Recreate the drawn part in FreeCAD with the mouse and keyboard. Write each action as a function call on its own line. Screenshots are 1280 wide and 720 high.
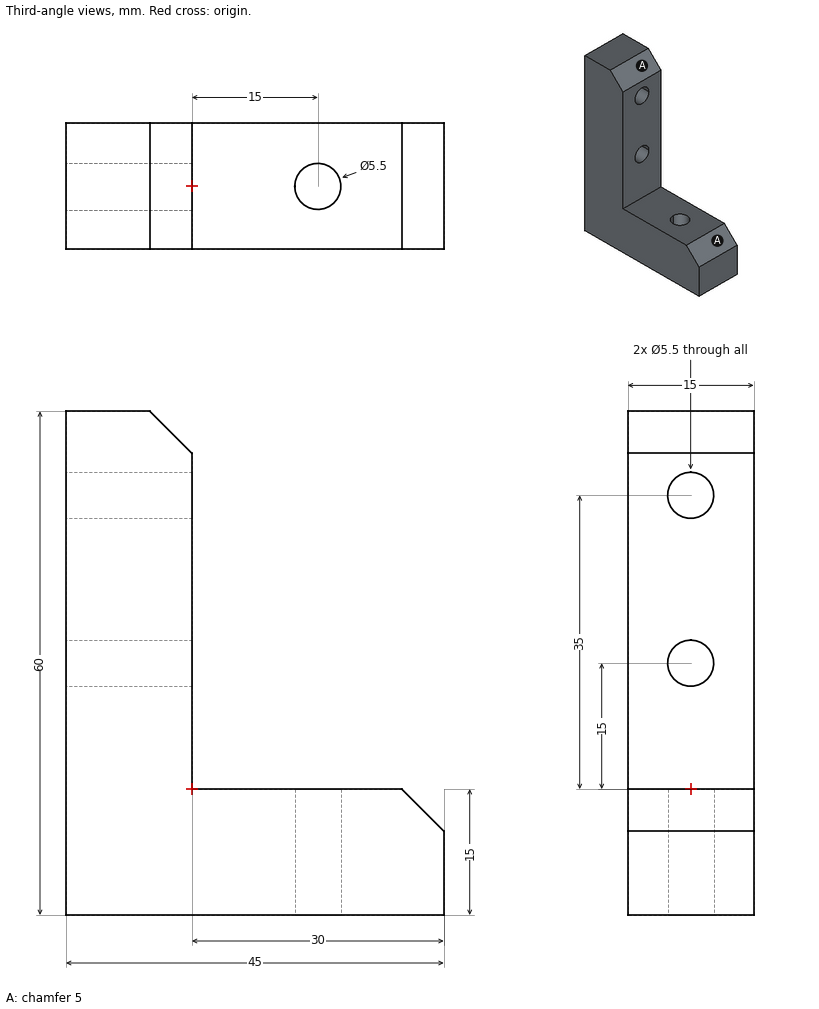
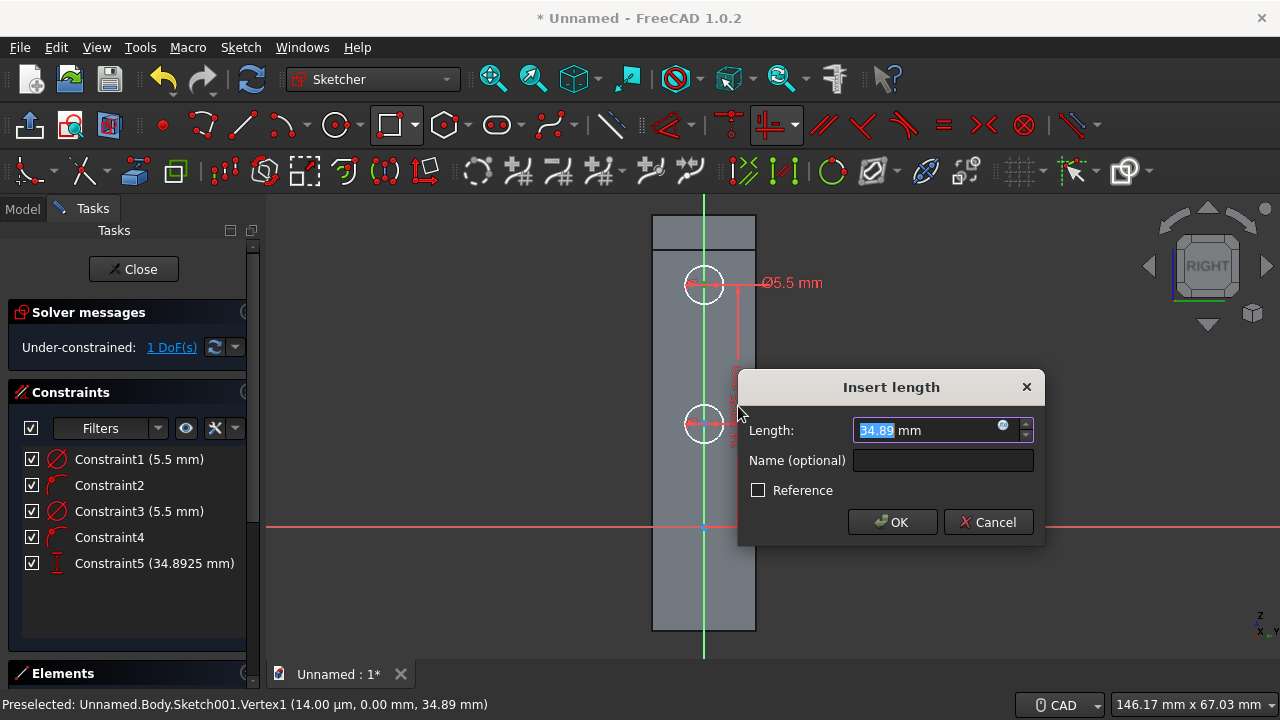
text(35)
key(Return)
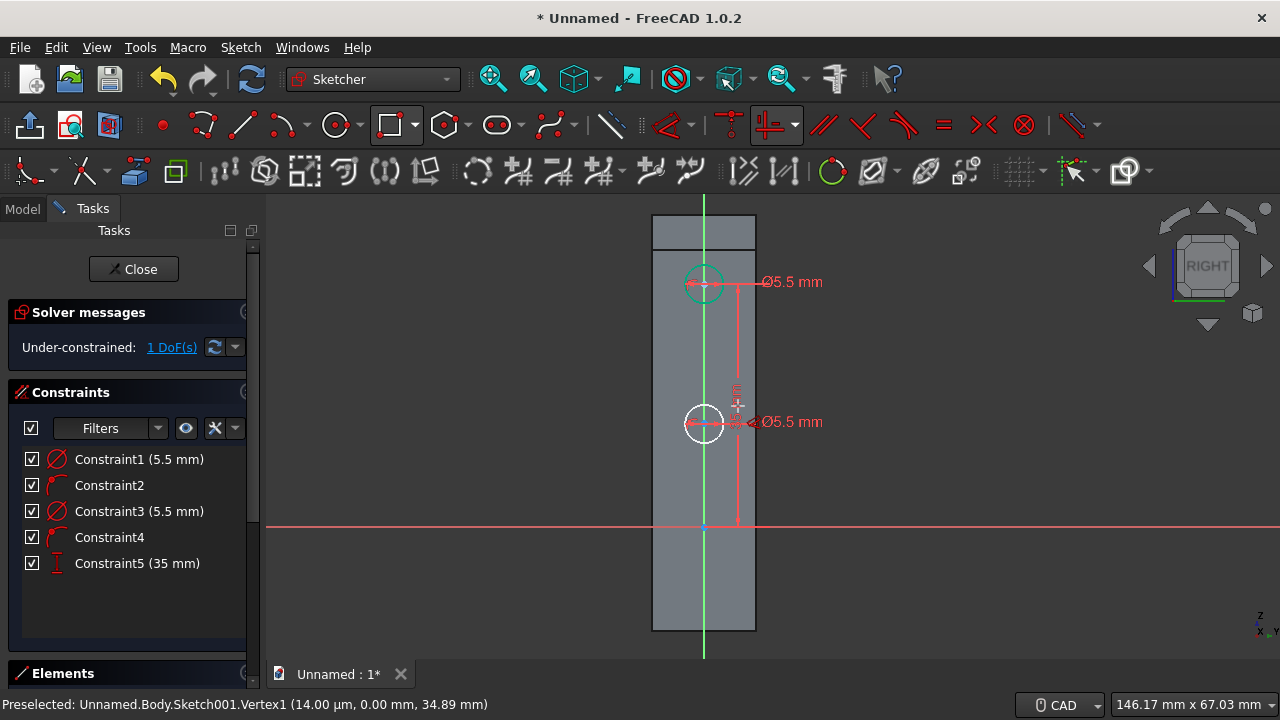
click(704, 424)
click(738, 476)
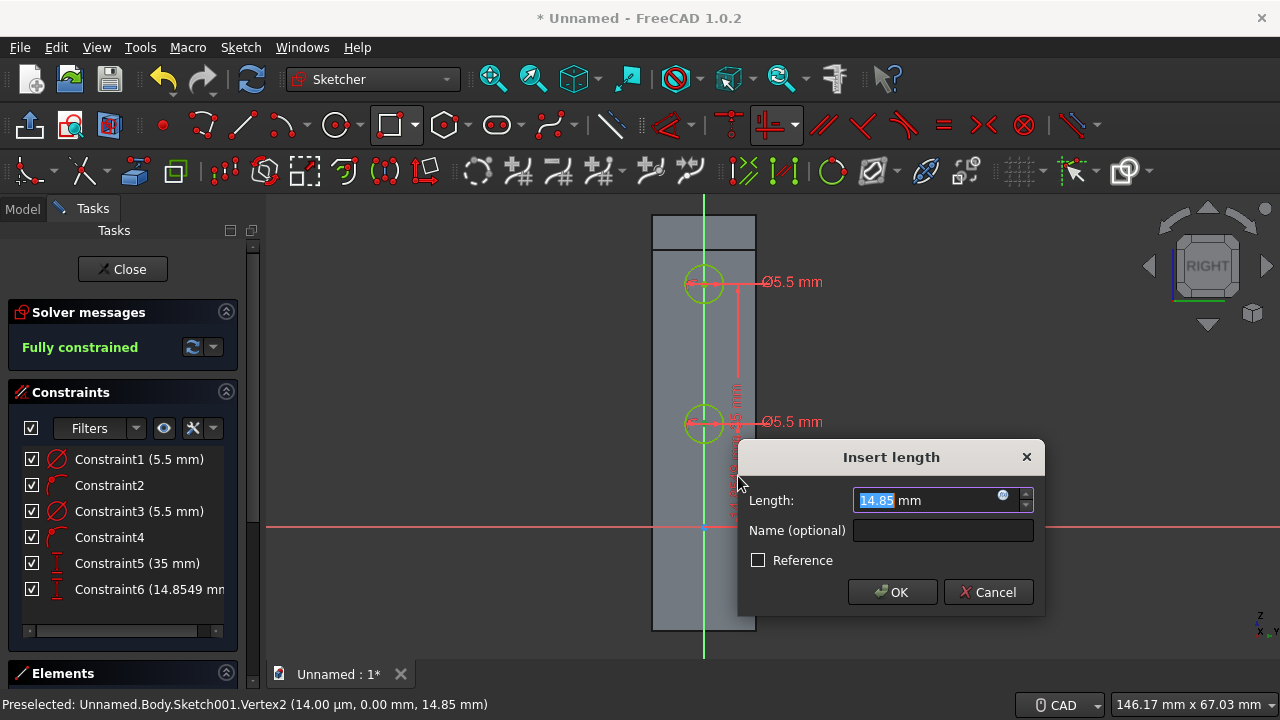
text(15)
key(Return)
key(Escape)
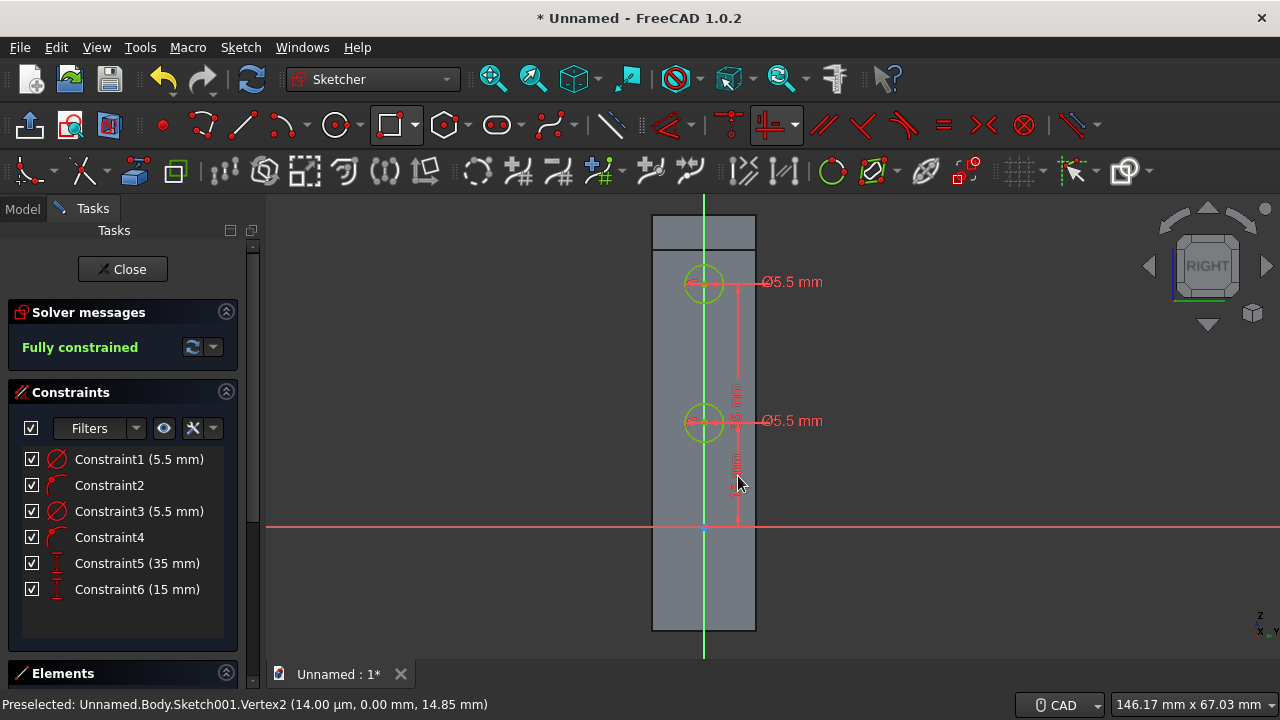
click(123, 269)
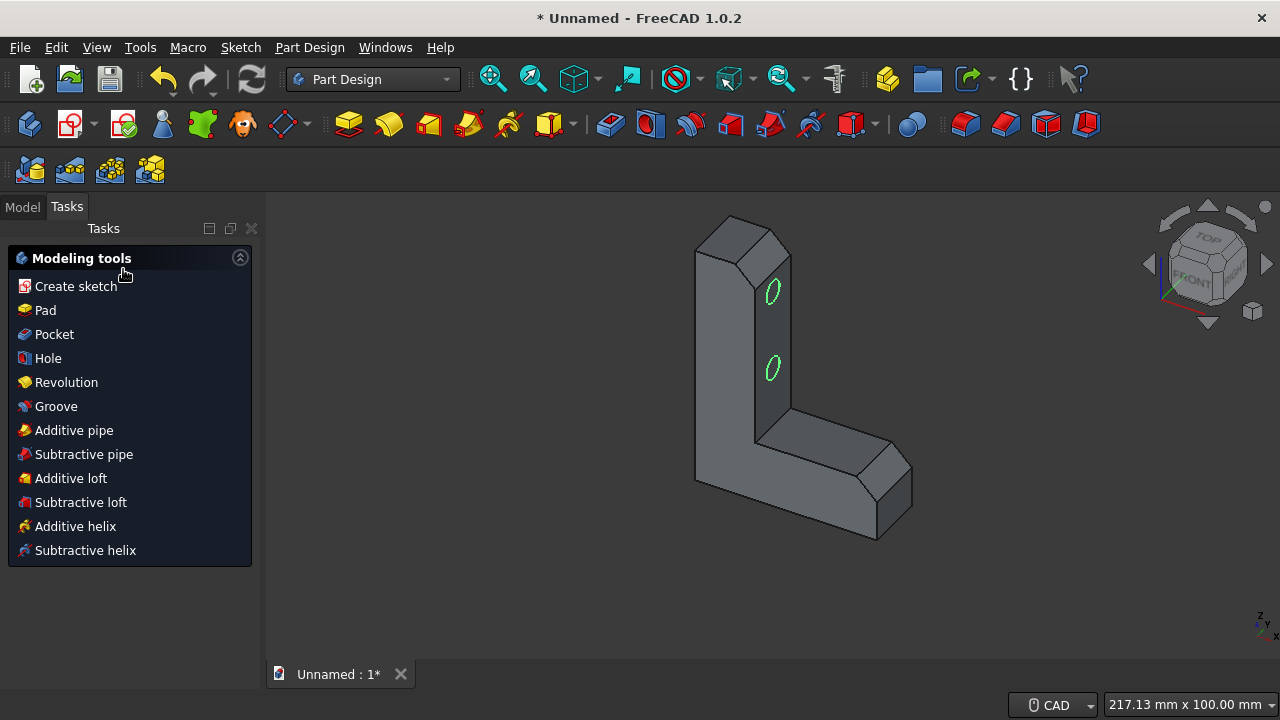
click(652, 124)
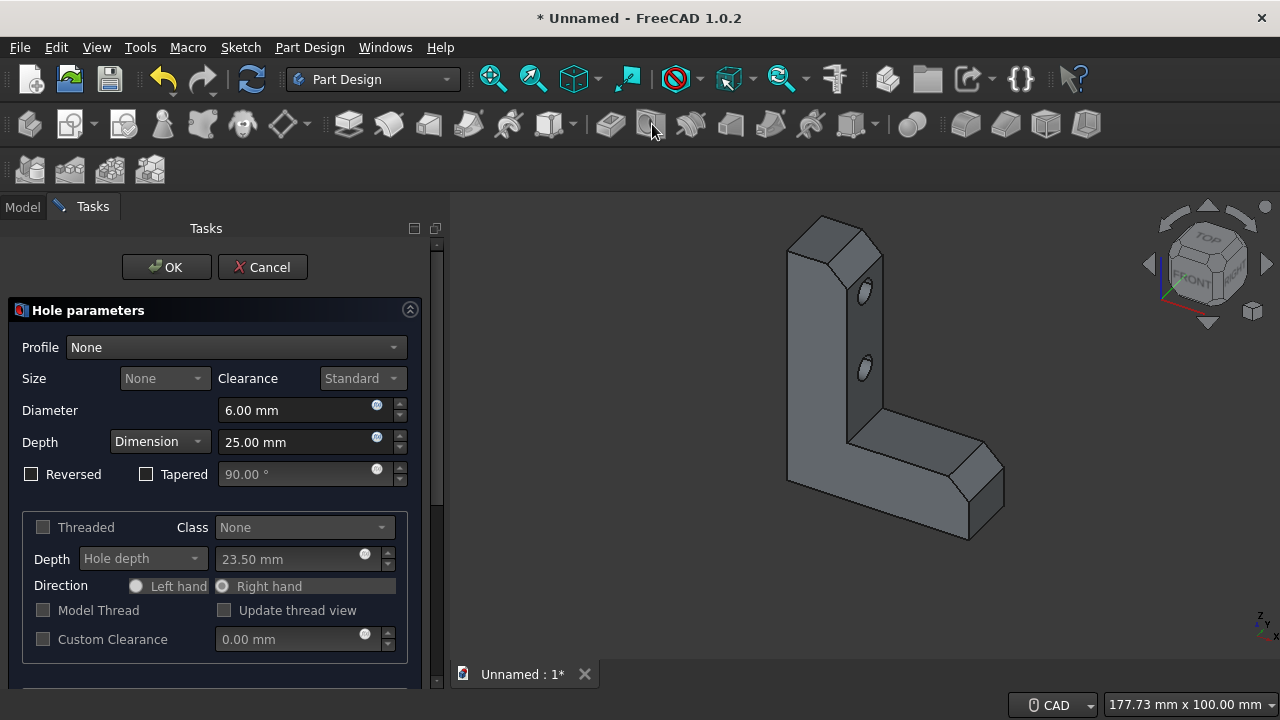
triple_click(305, 410)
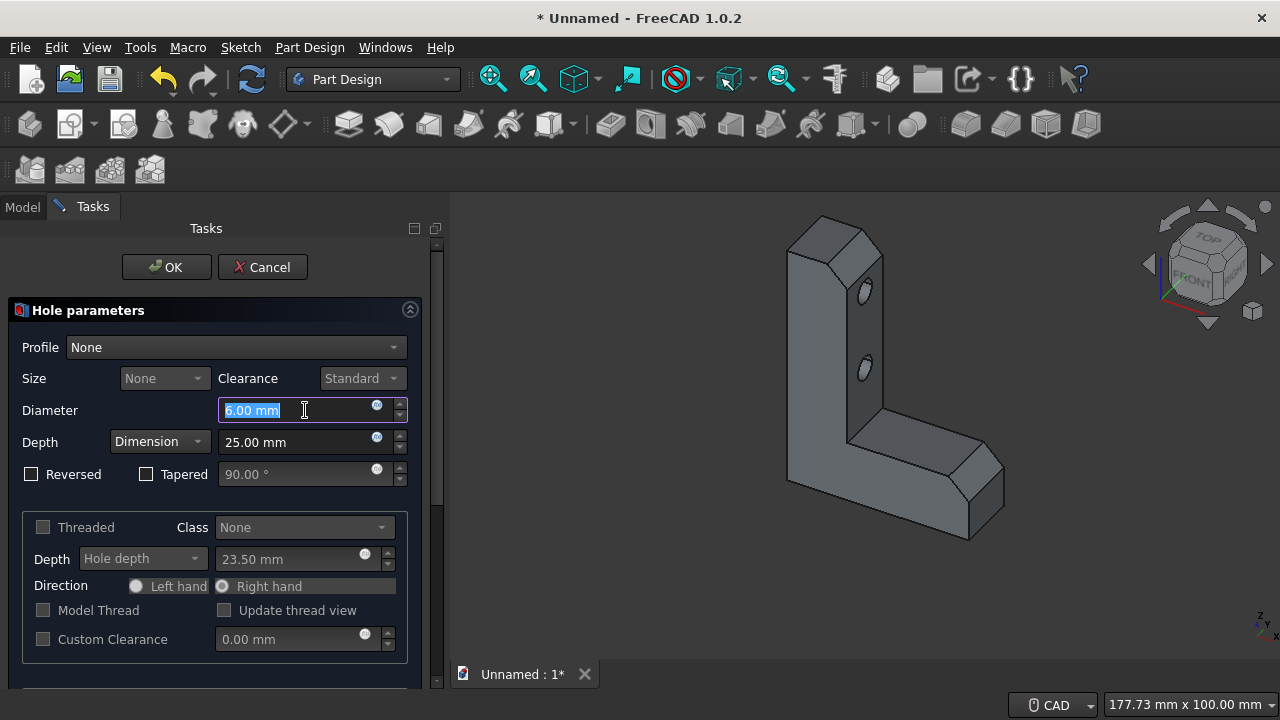
text(5.5)
key(Tab)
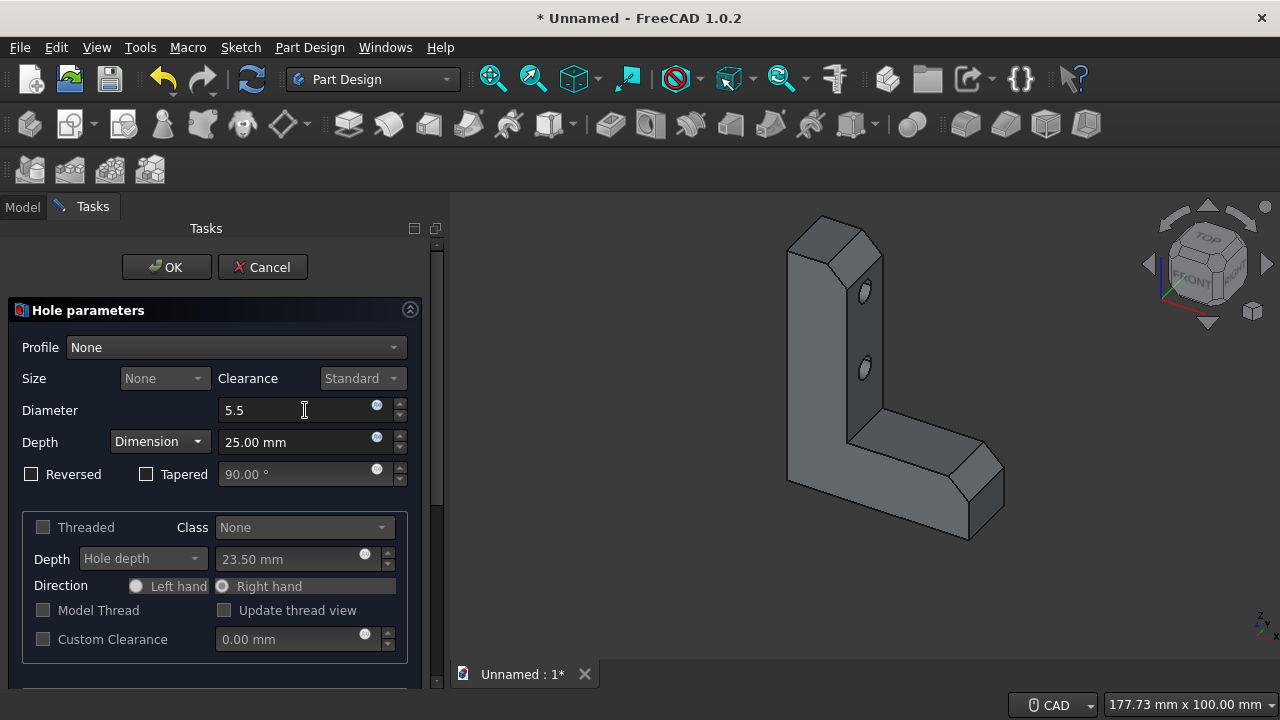
click(161, 442)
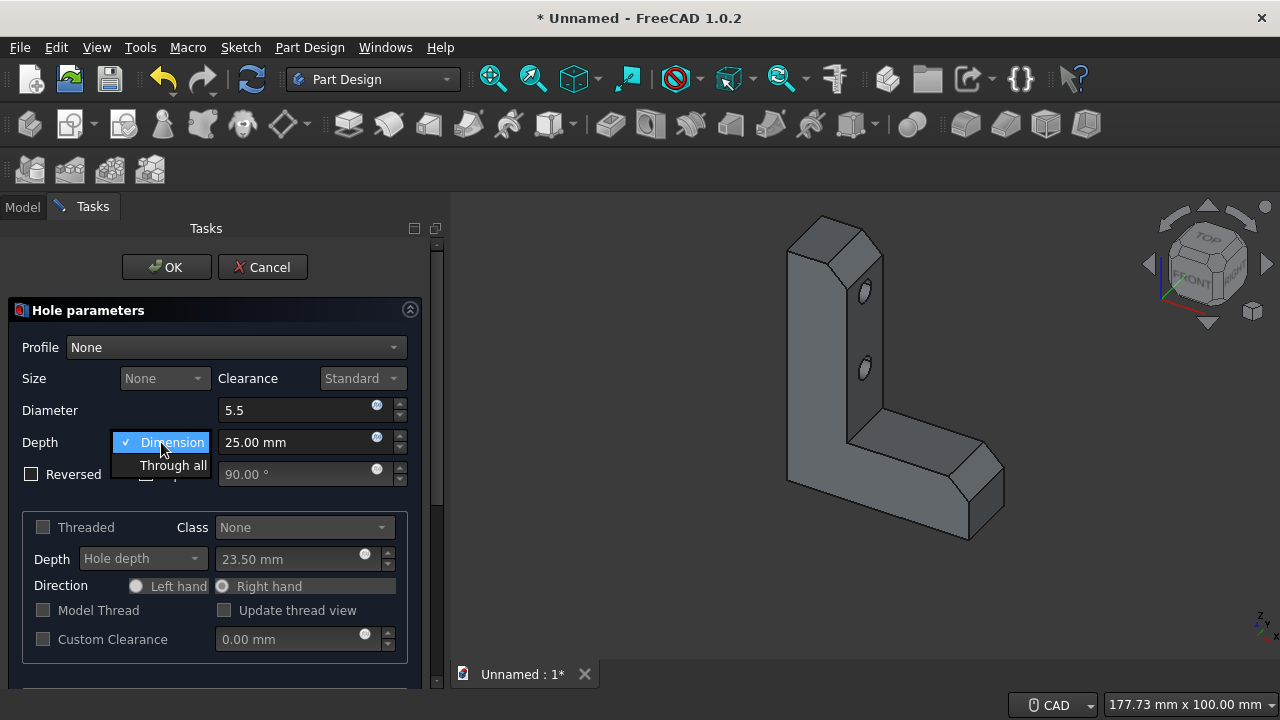
click(160, 466)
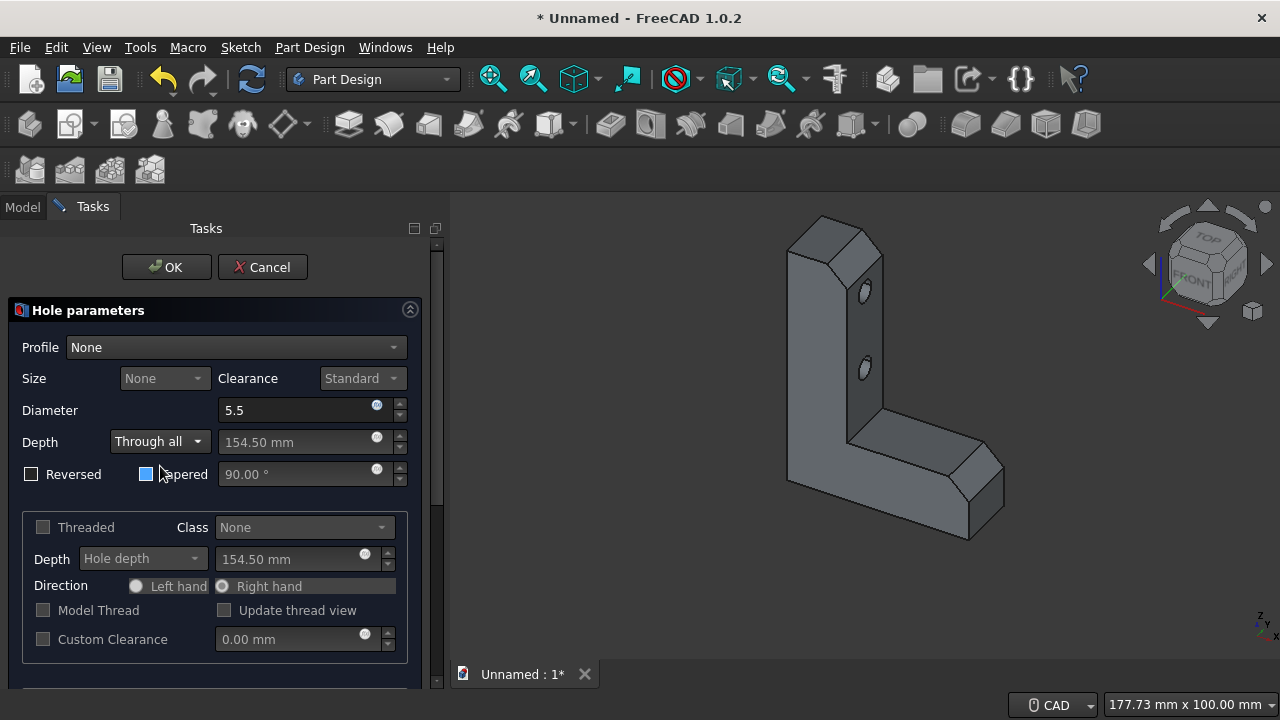
click(167, 267)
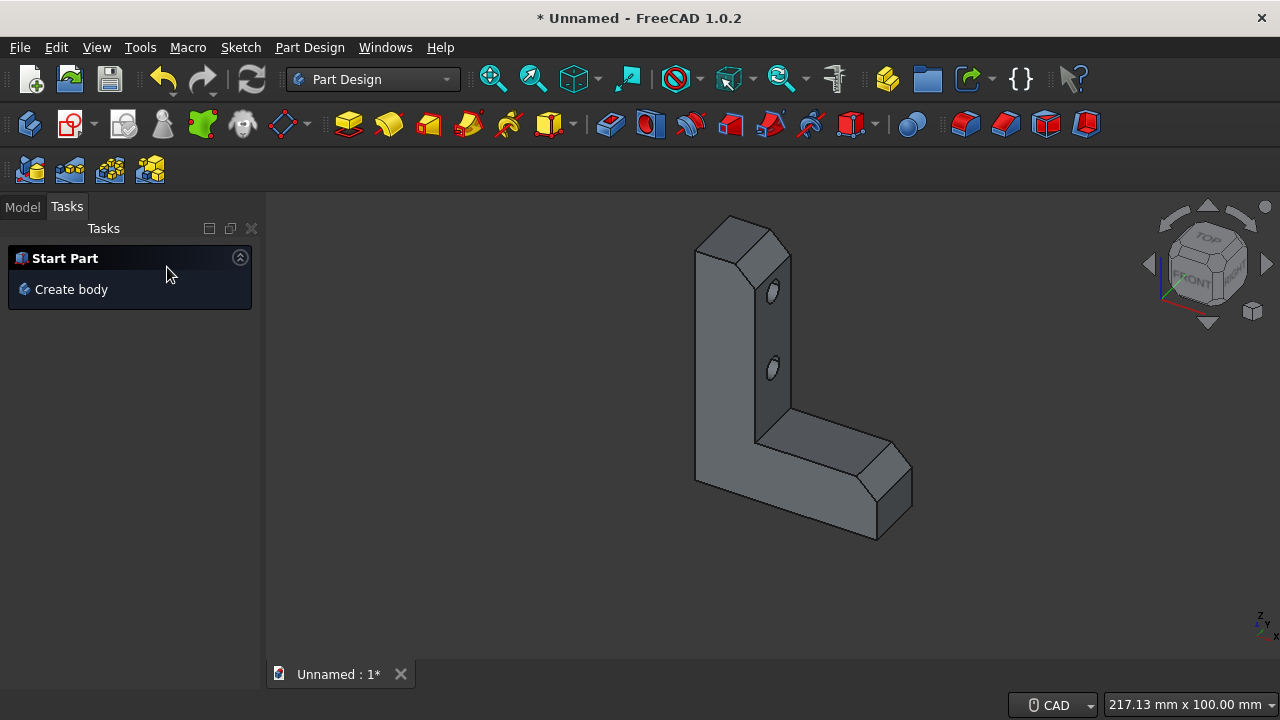
click(838, 446)